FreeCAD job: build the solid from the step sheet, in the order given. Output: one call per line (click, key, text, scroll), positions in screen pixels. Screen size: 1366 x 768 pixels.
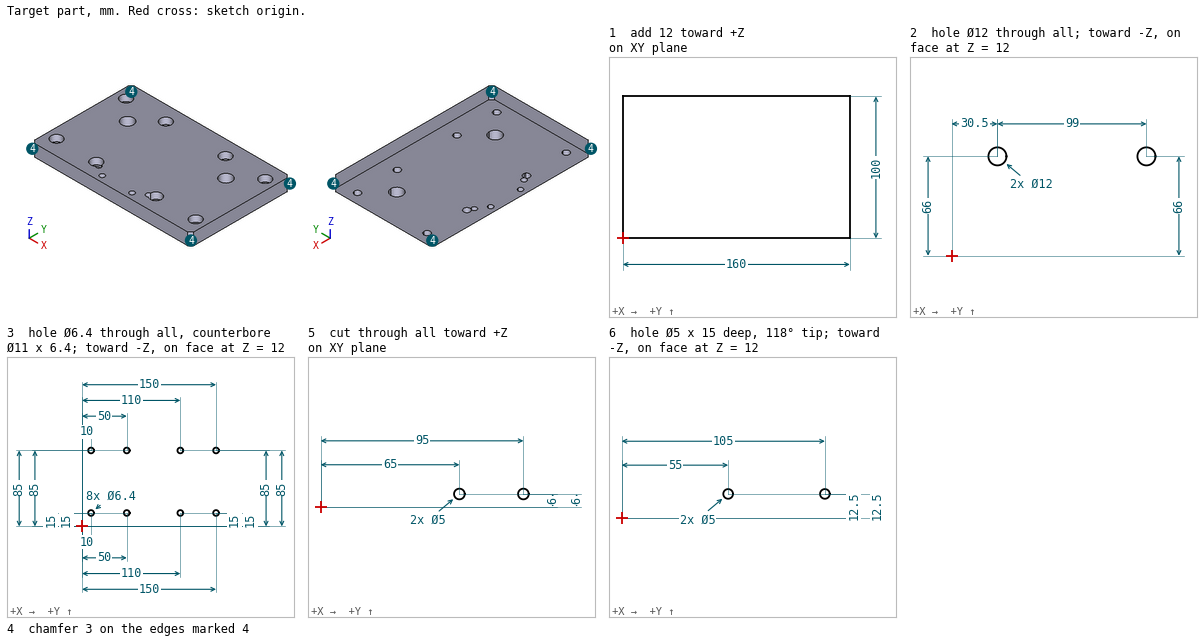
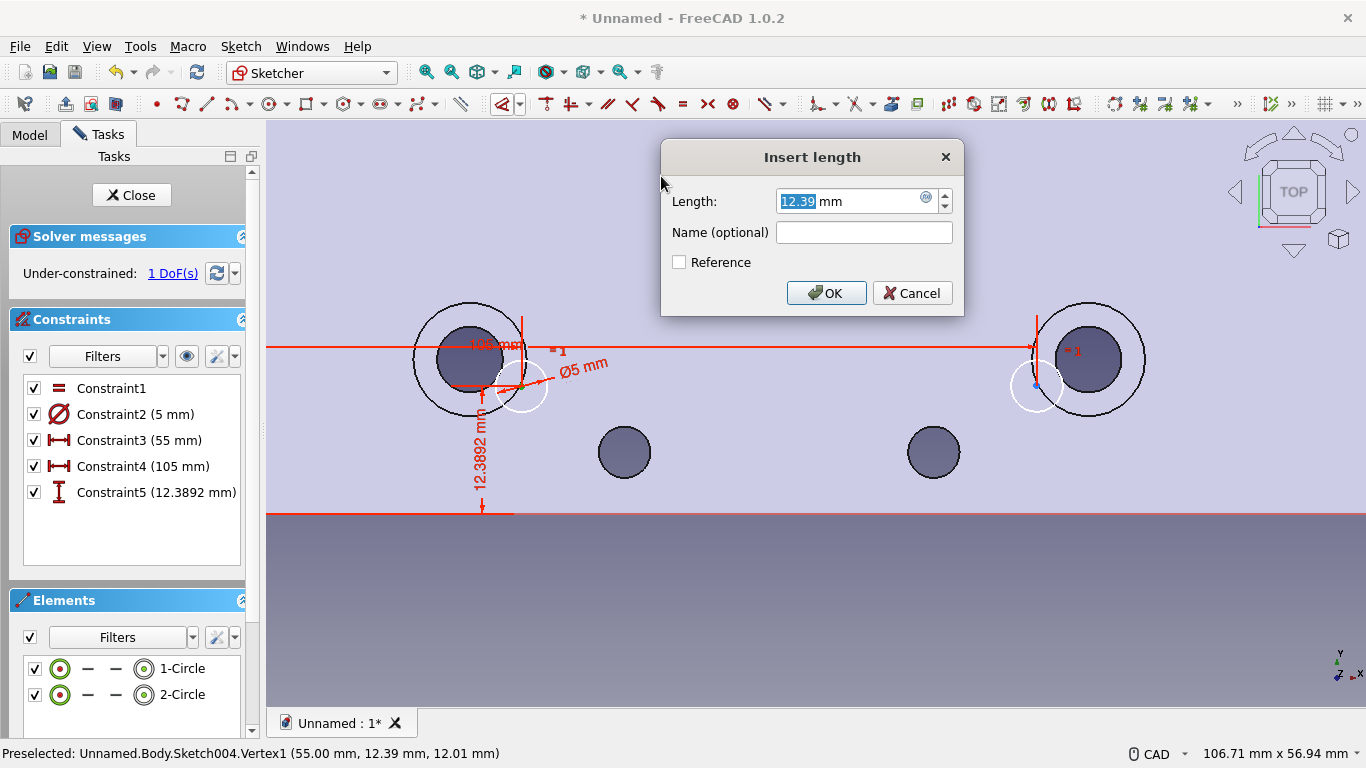
text(12.5)
key(Return)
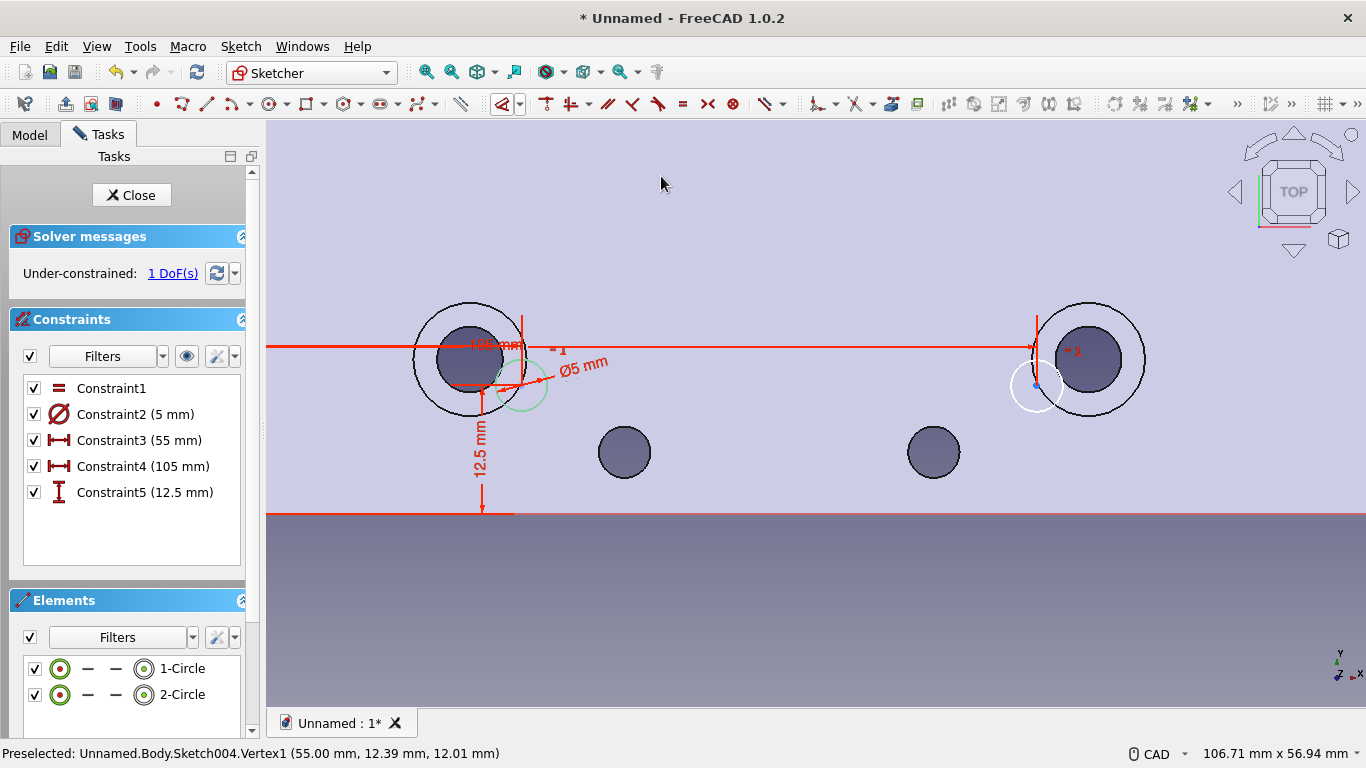
click(1037, 386)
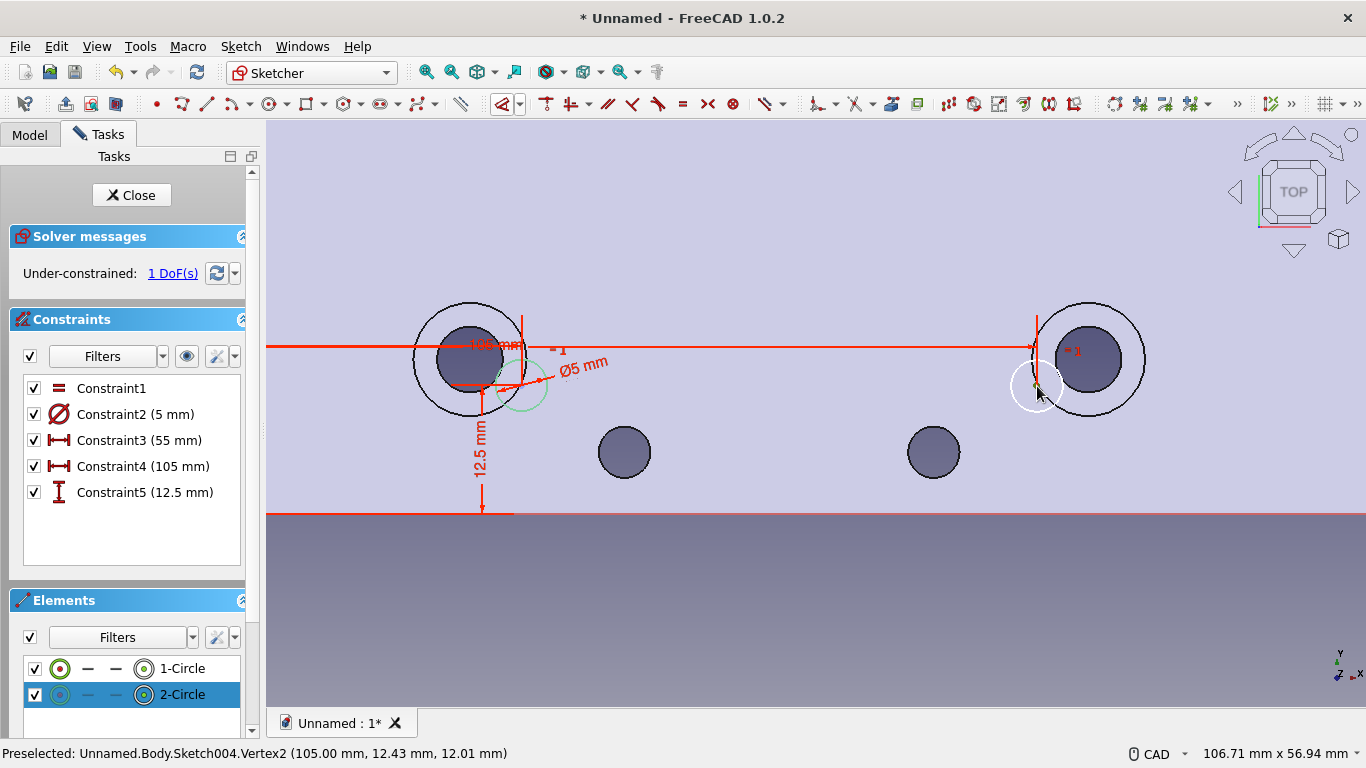
key(i)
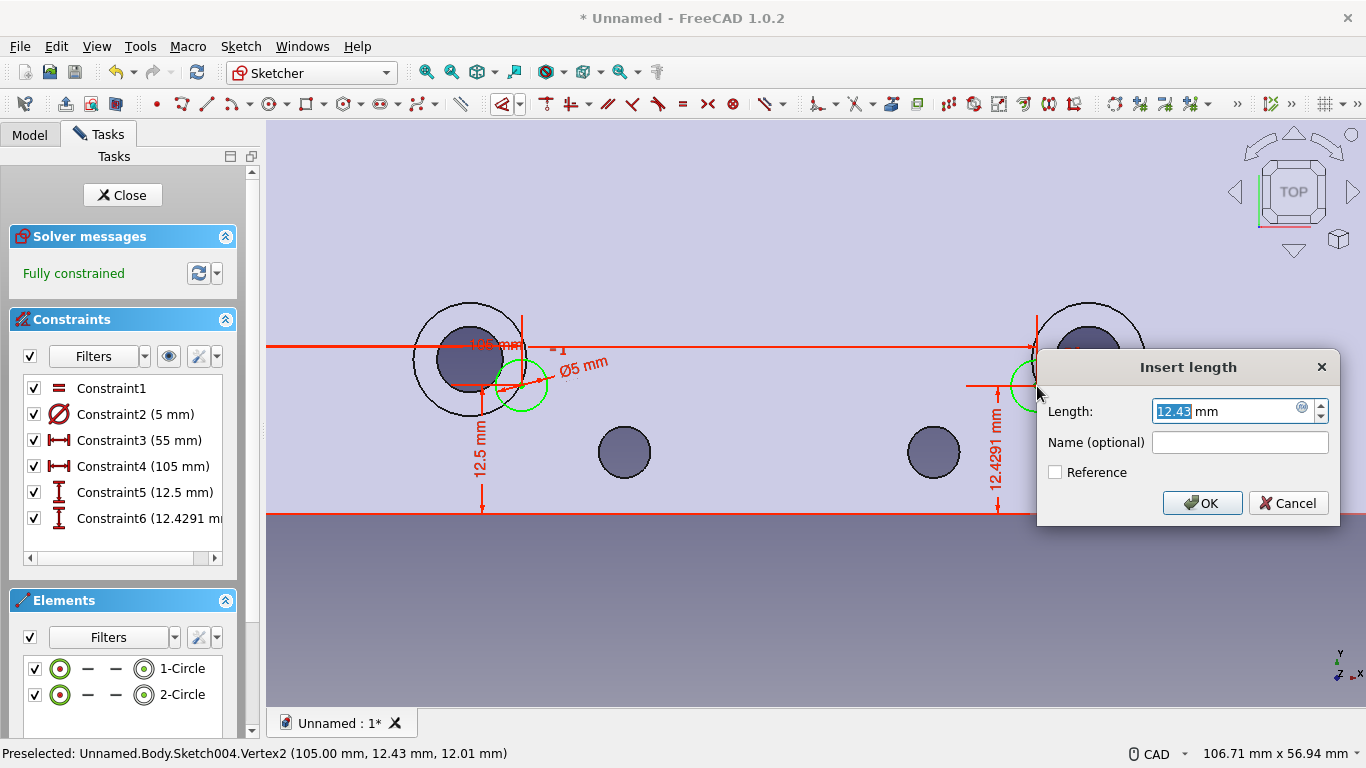
text(12.5)
key(Return)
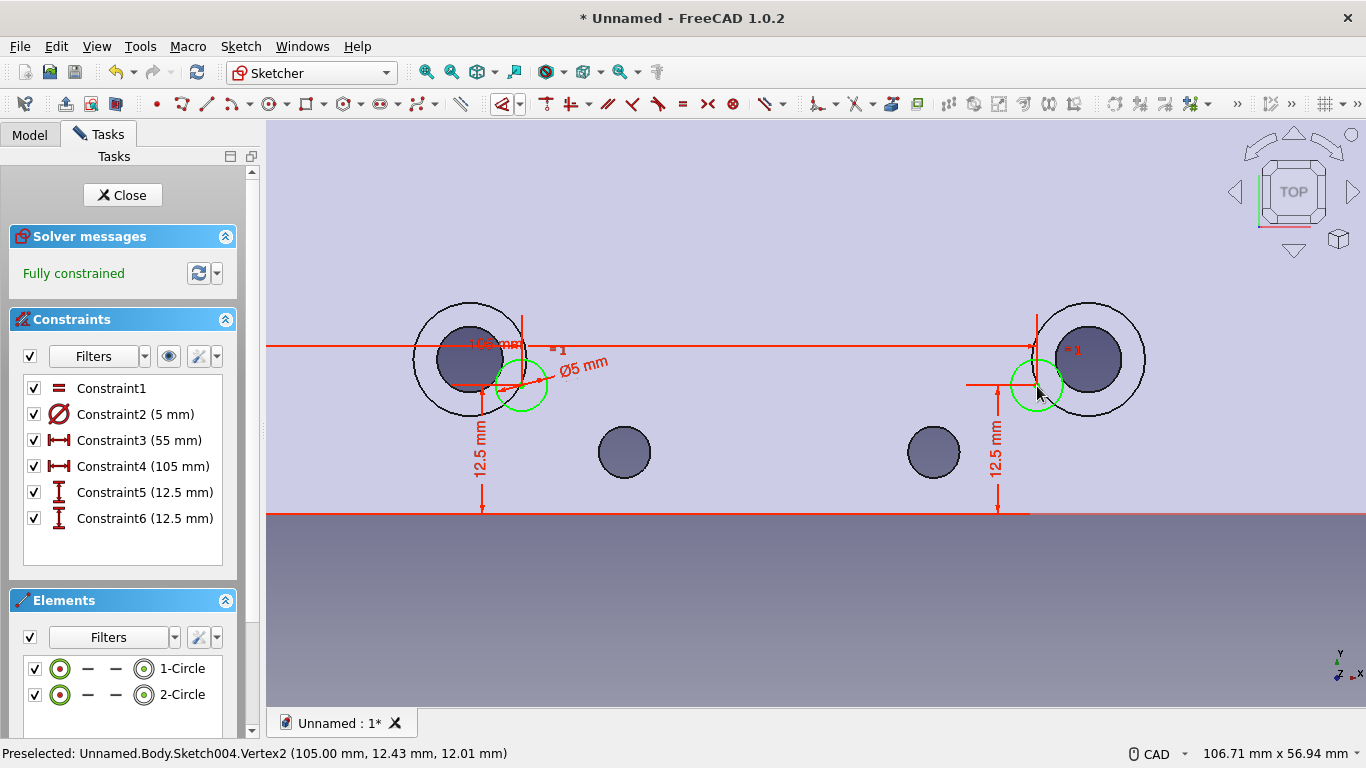
click(123, 195)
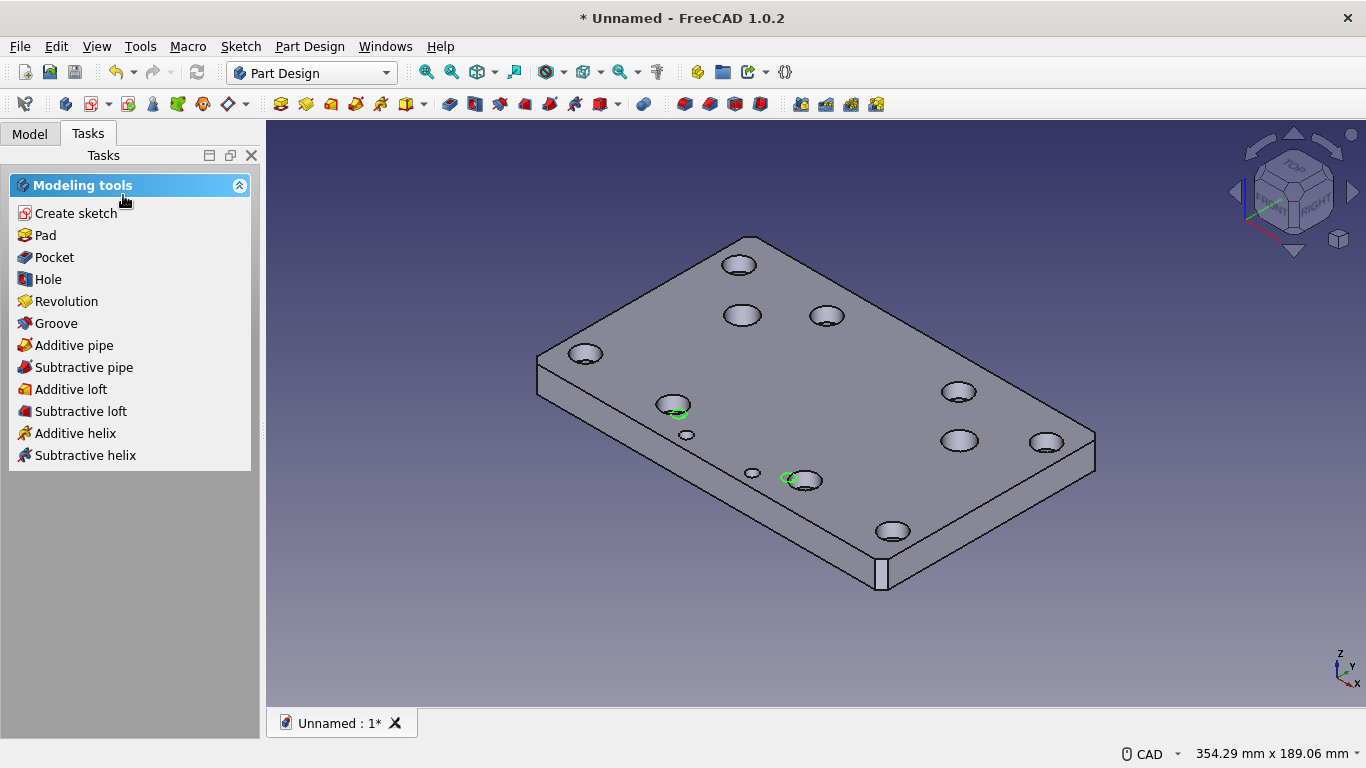
click(475, 104)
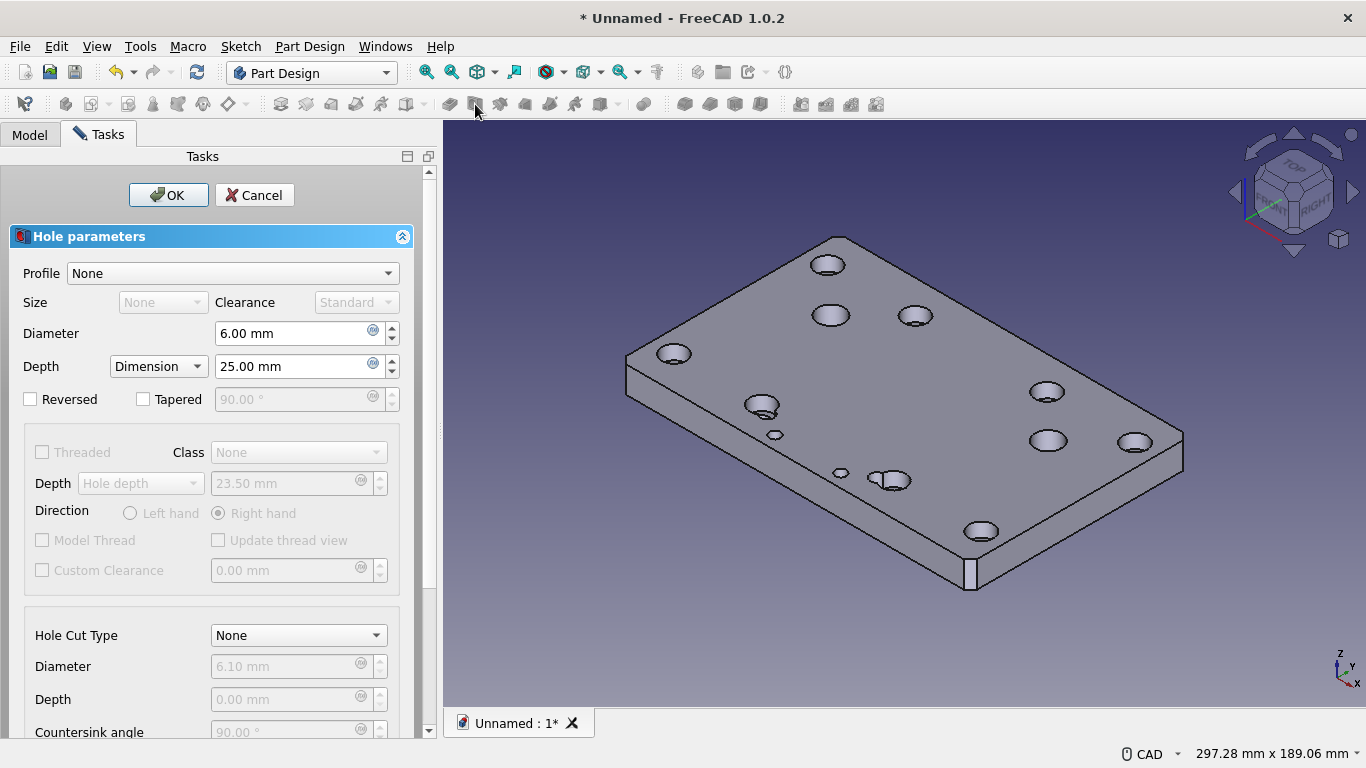
triple_click(300, 334)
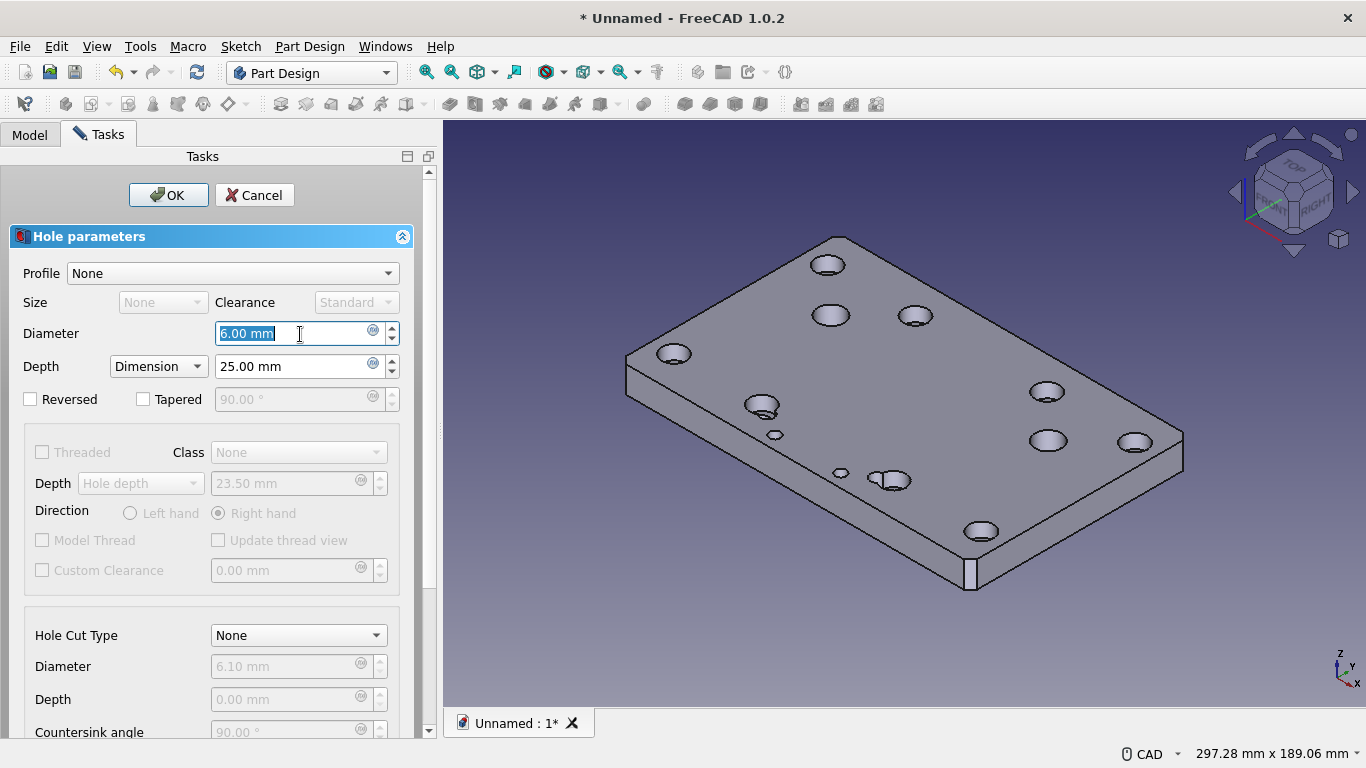
text(5)
key(Tab)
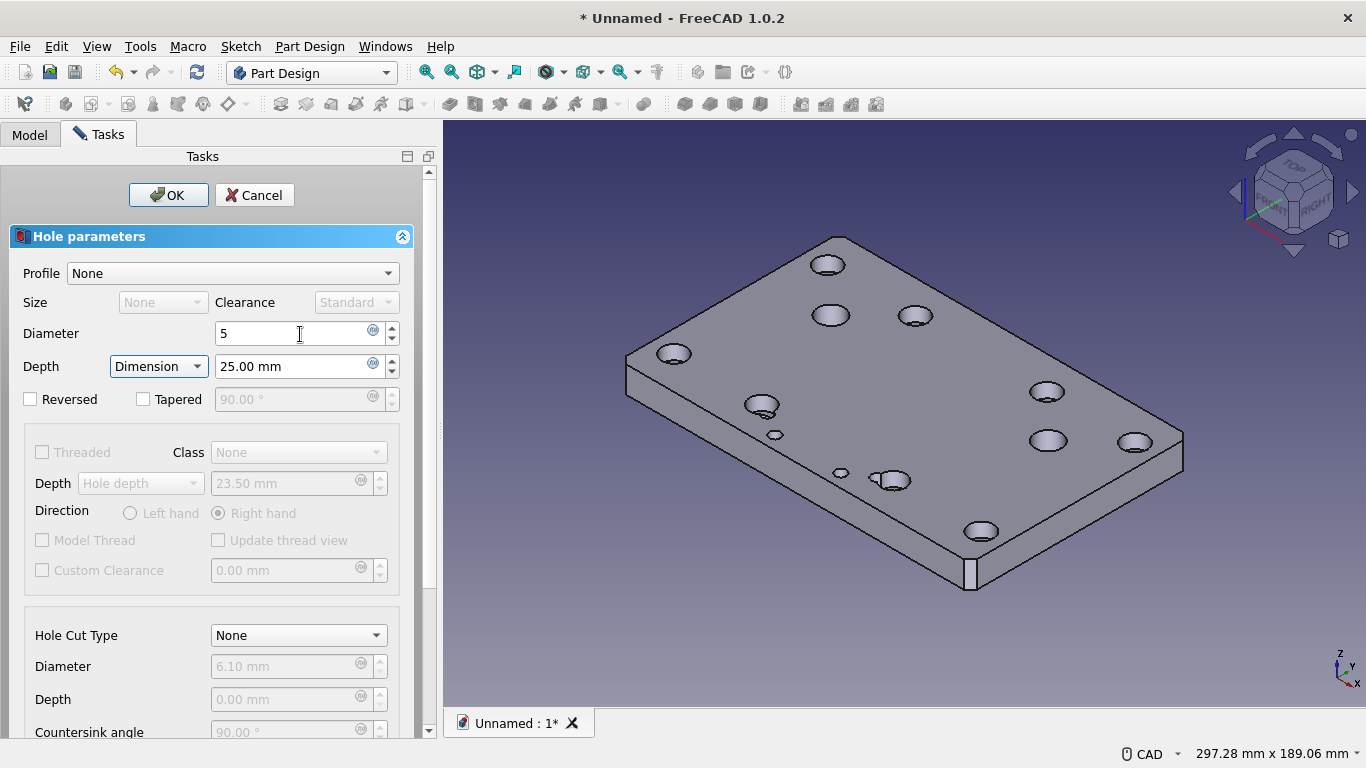
triple_click(300, 366)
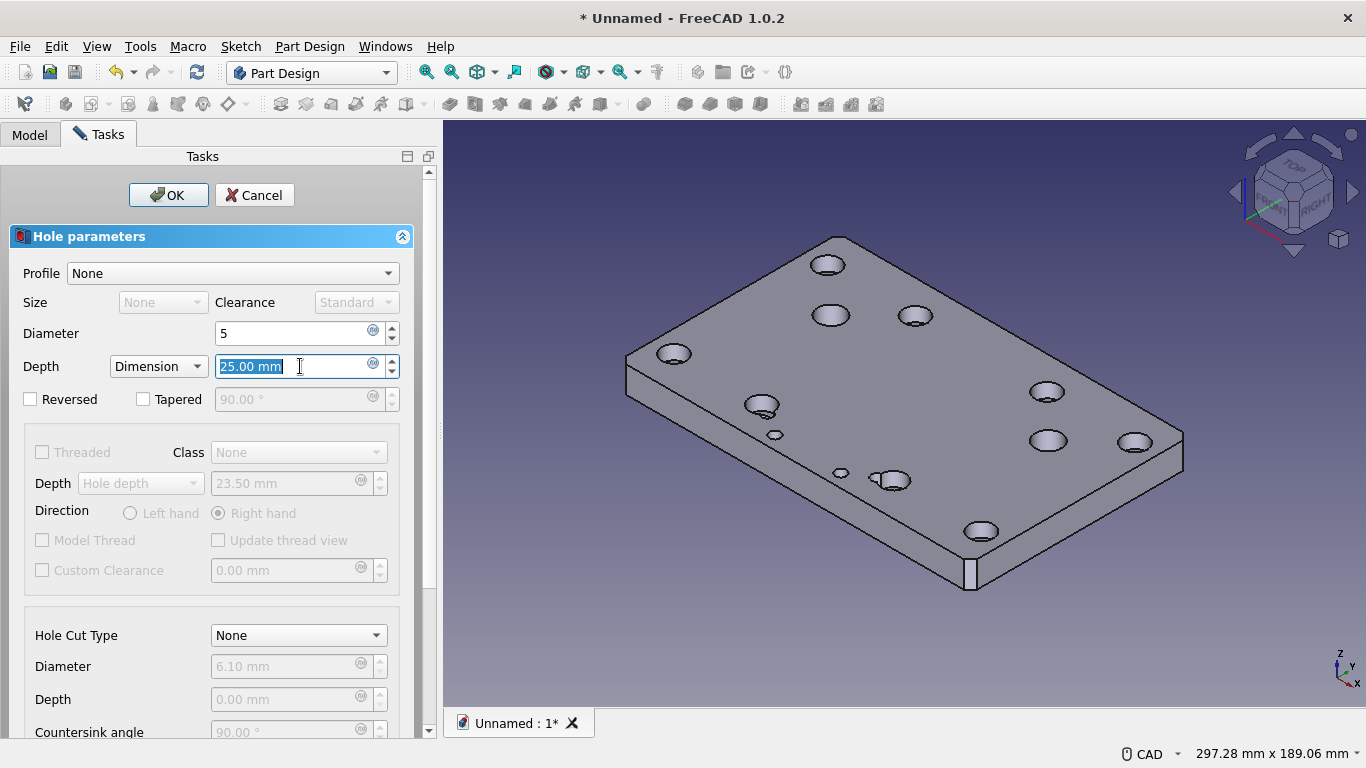
text(15)
key(Tab)